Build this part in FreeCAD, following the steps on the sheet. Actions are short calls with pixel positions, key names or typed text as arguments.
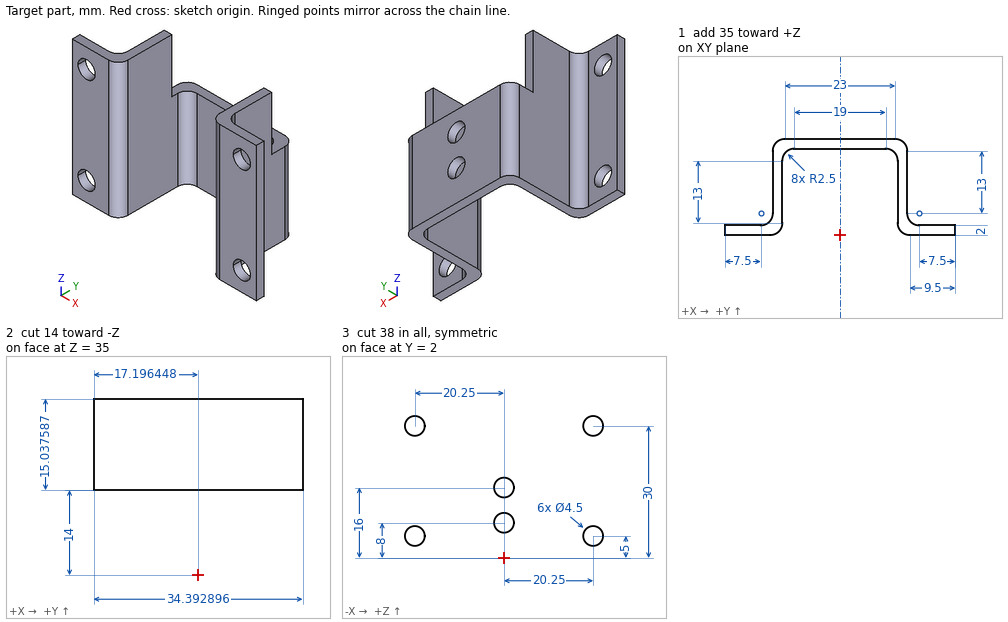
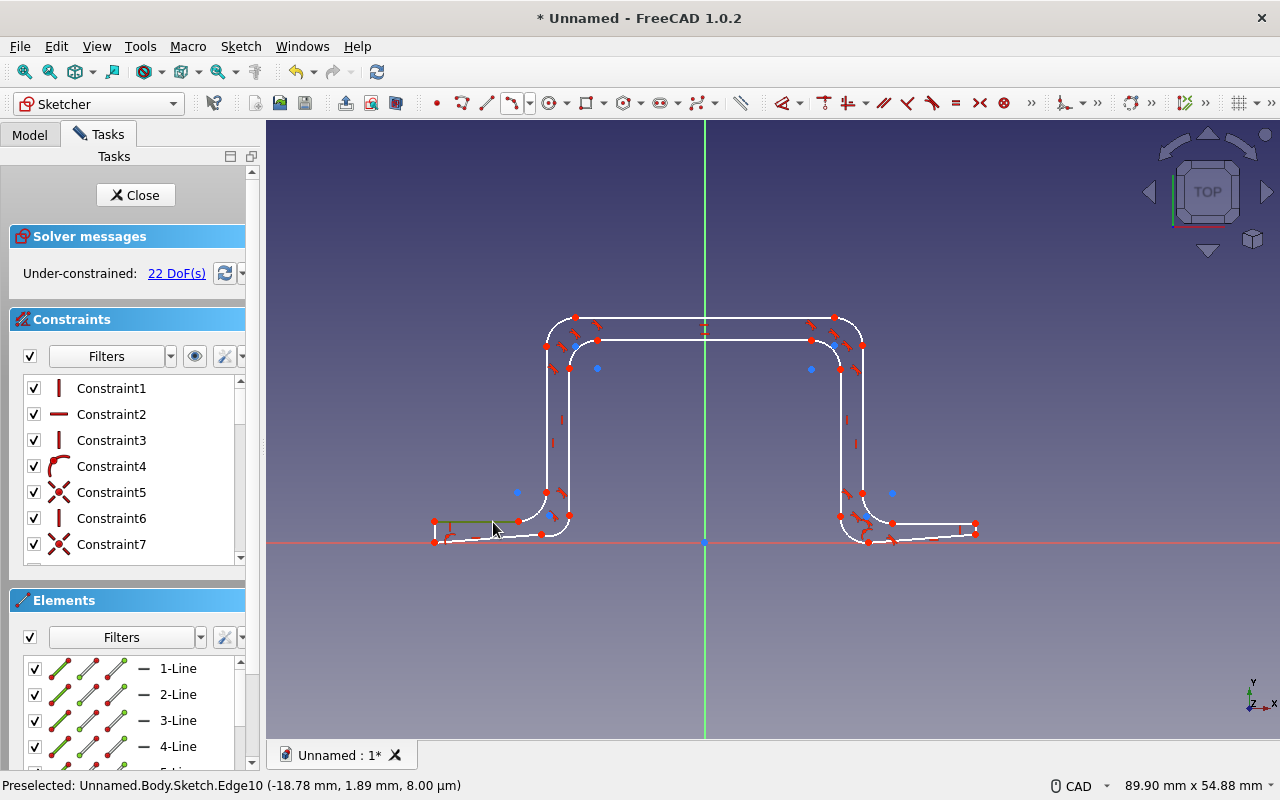
click(531, 518)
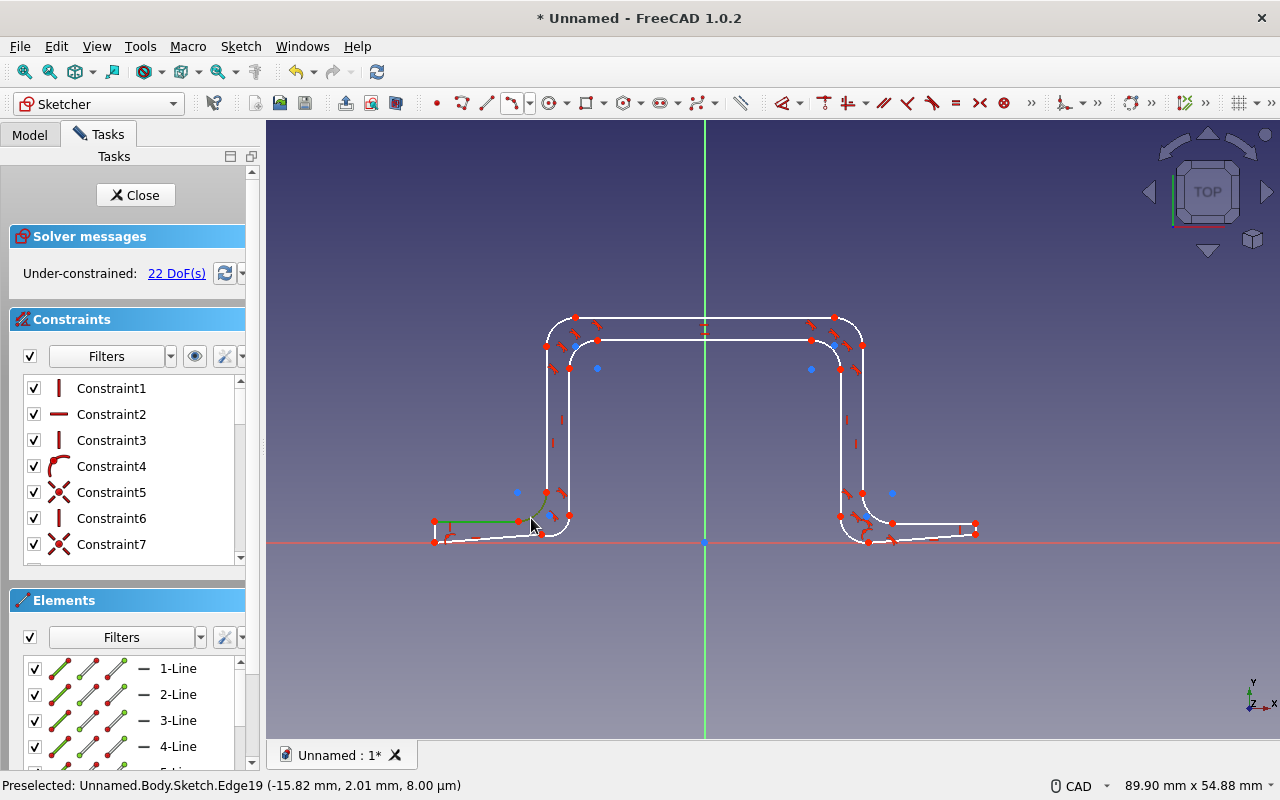
click(932, 104)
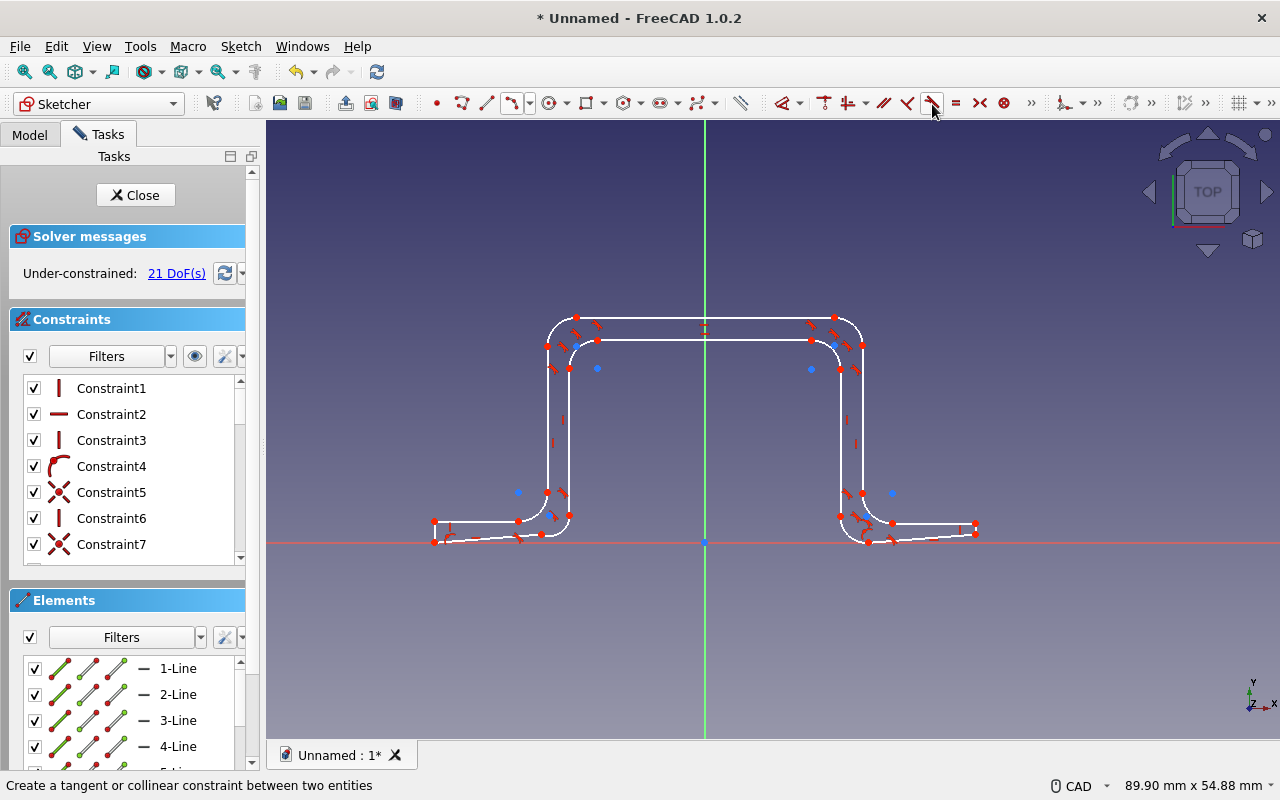
click(467, 540)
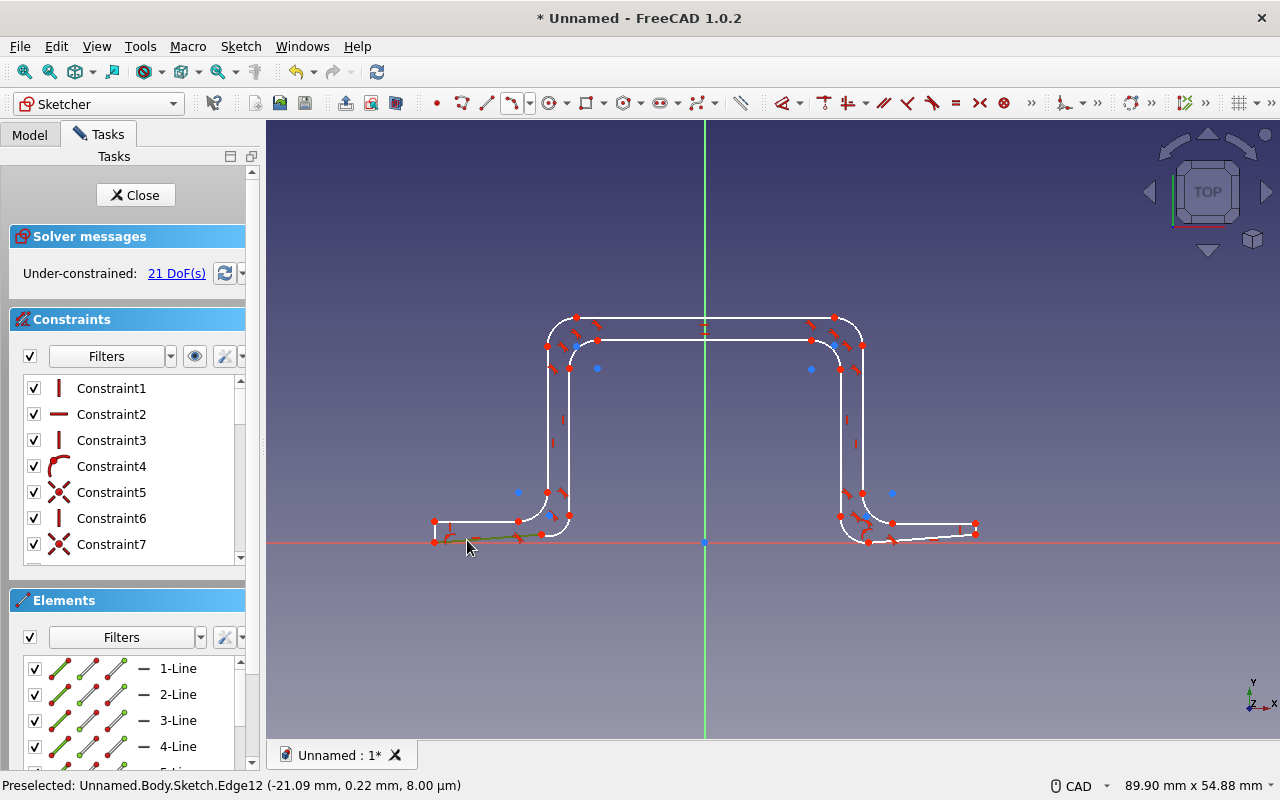
click(566, 527)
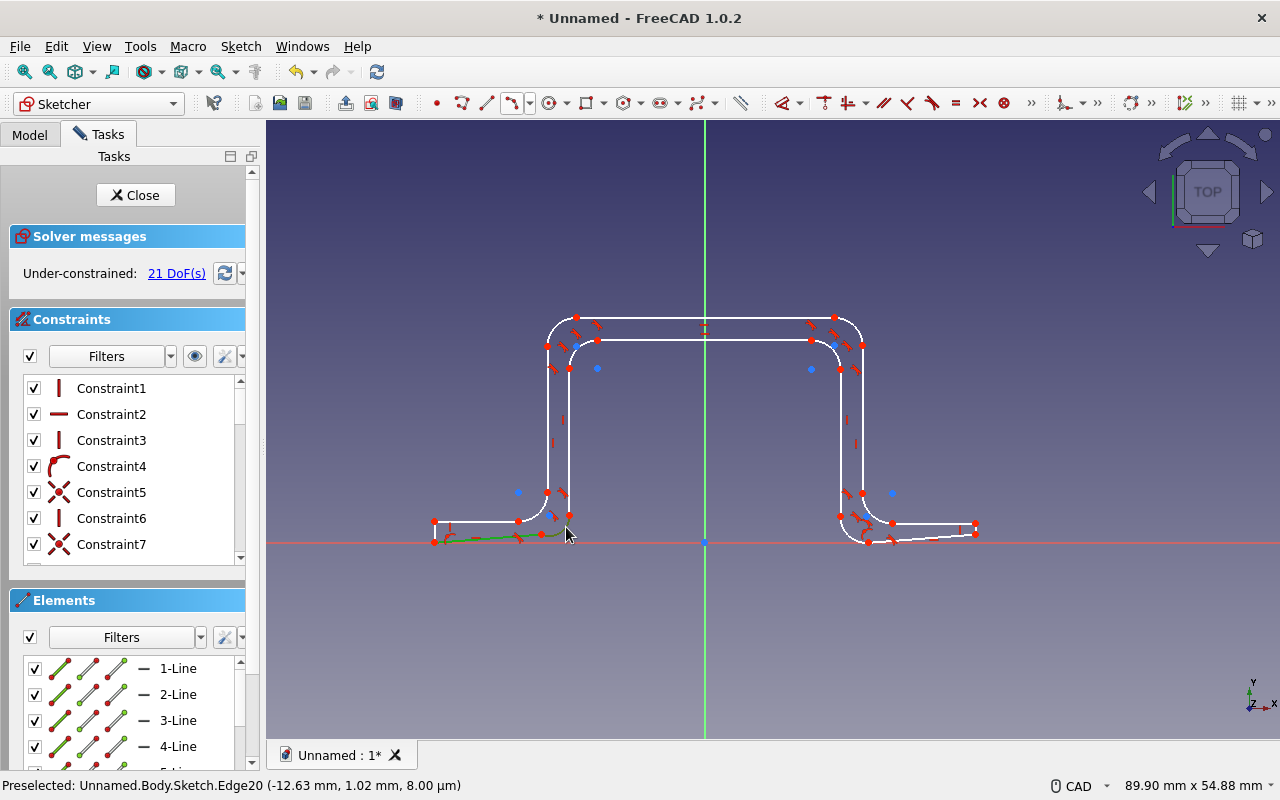
click(932, 104)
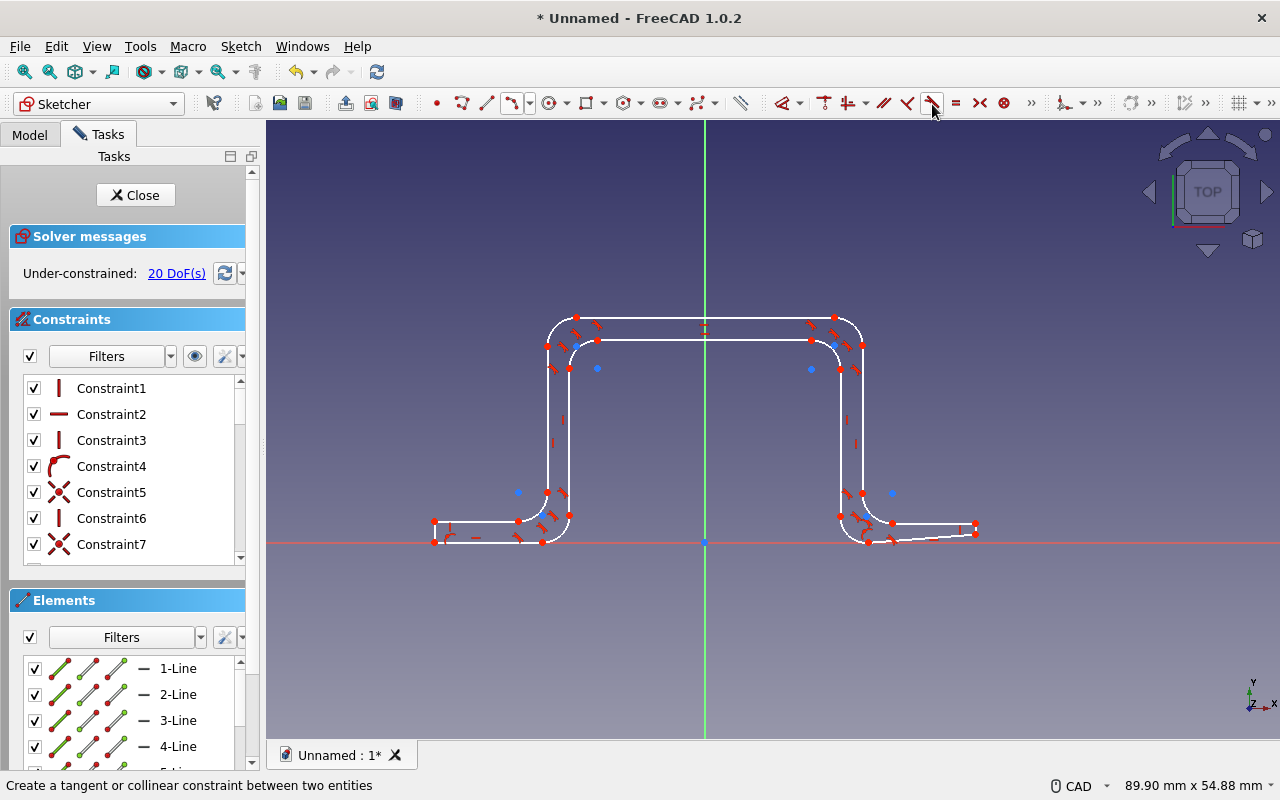
click(901, 540)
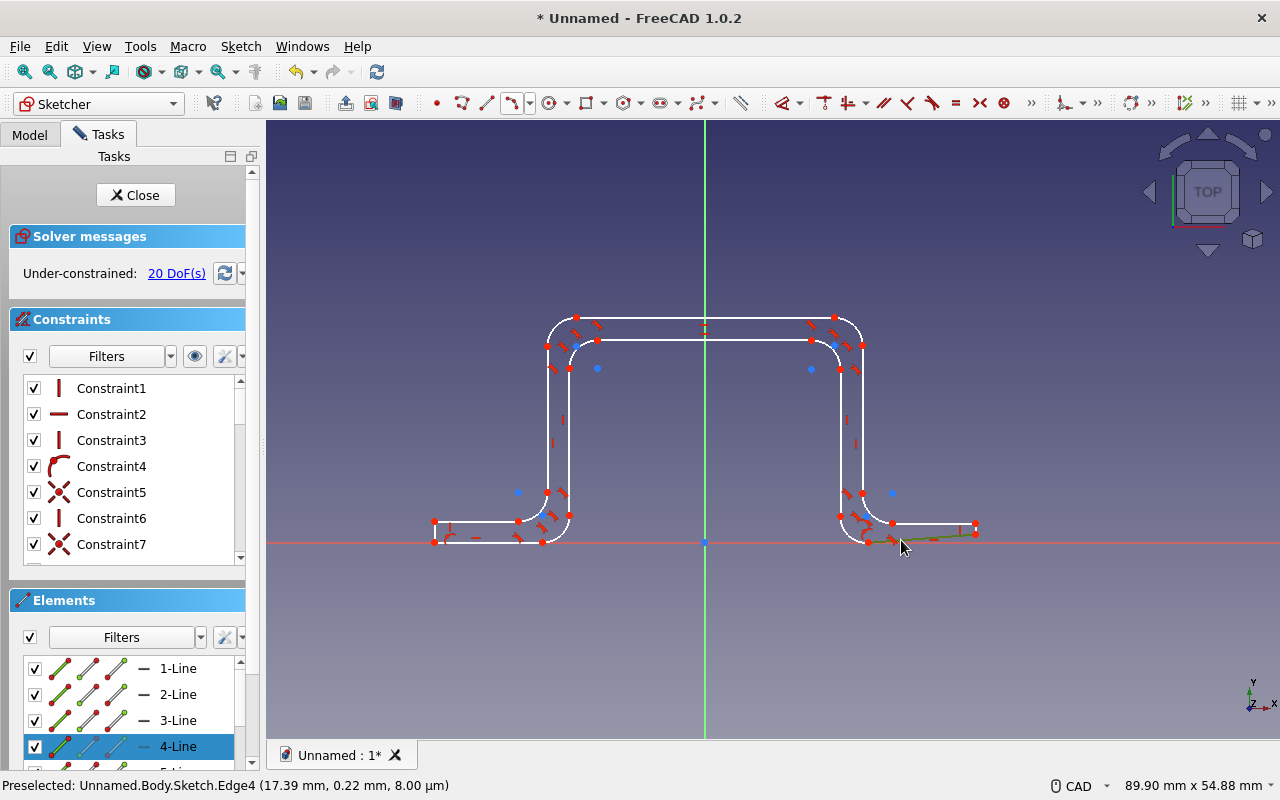
click(866, 104)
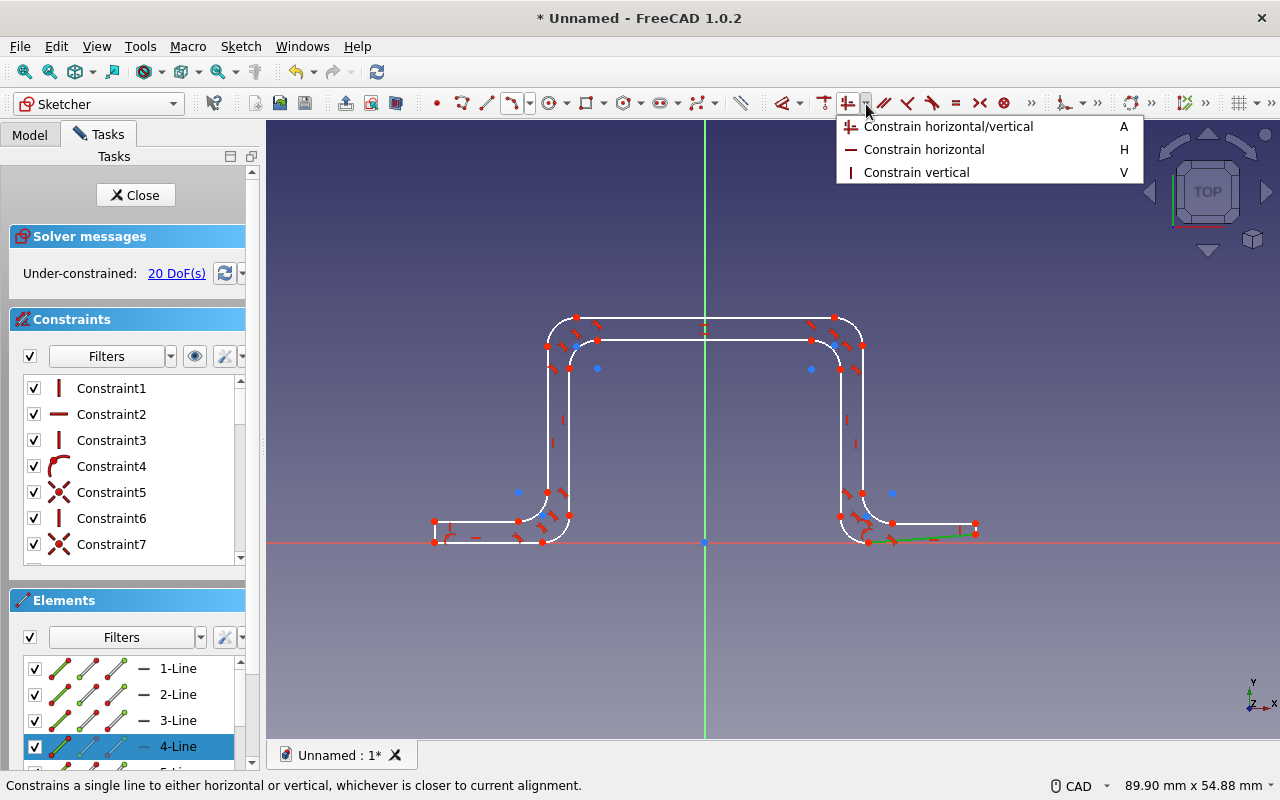
click(990, 150)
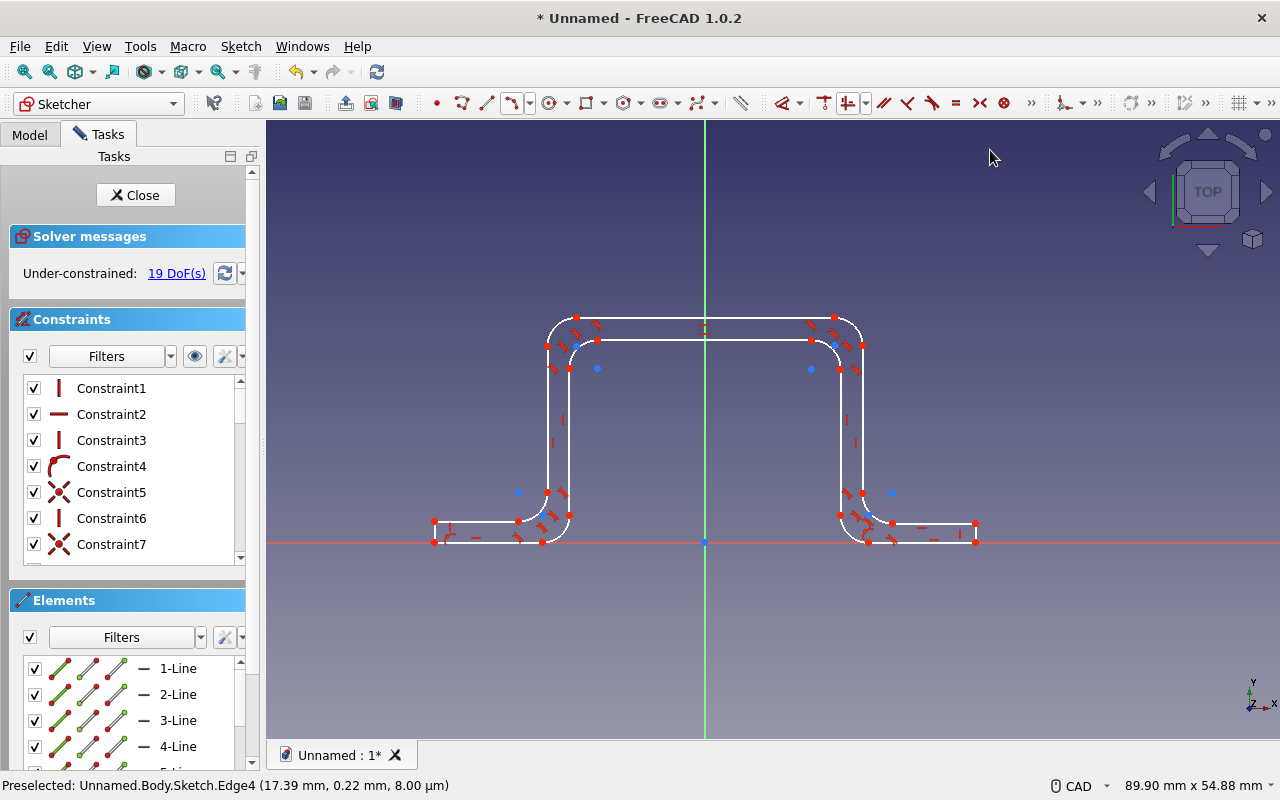
click(467, 543)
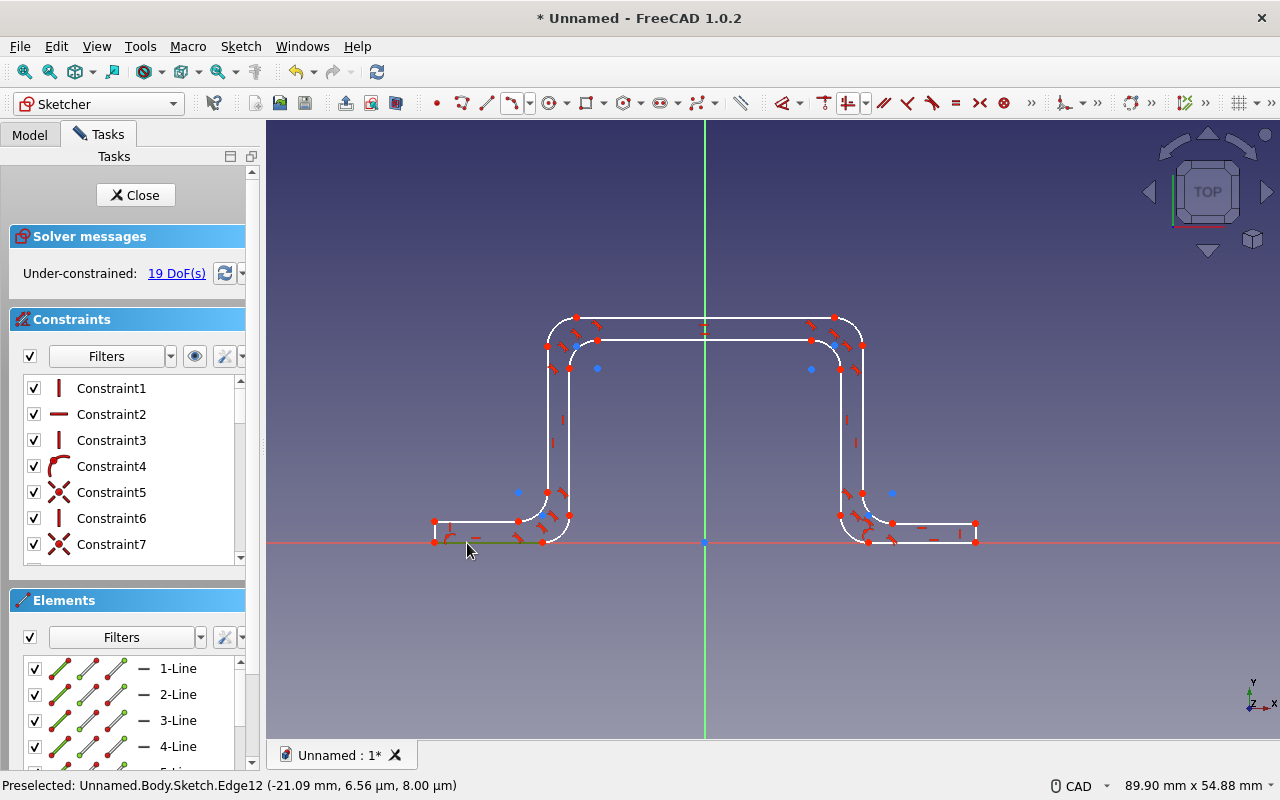
key(h)